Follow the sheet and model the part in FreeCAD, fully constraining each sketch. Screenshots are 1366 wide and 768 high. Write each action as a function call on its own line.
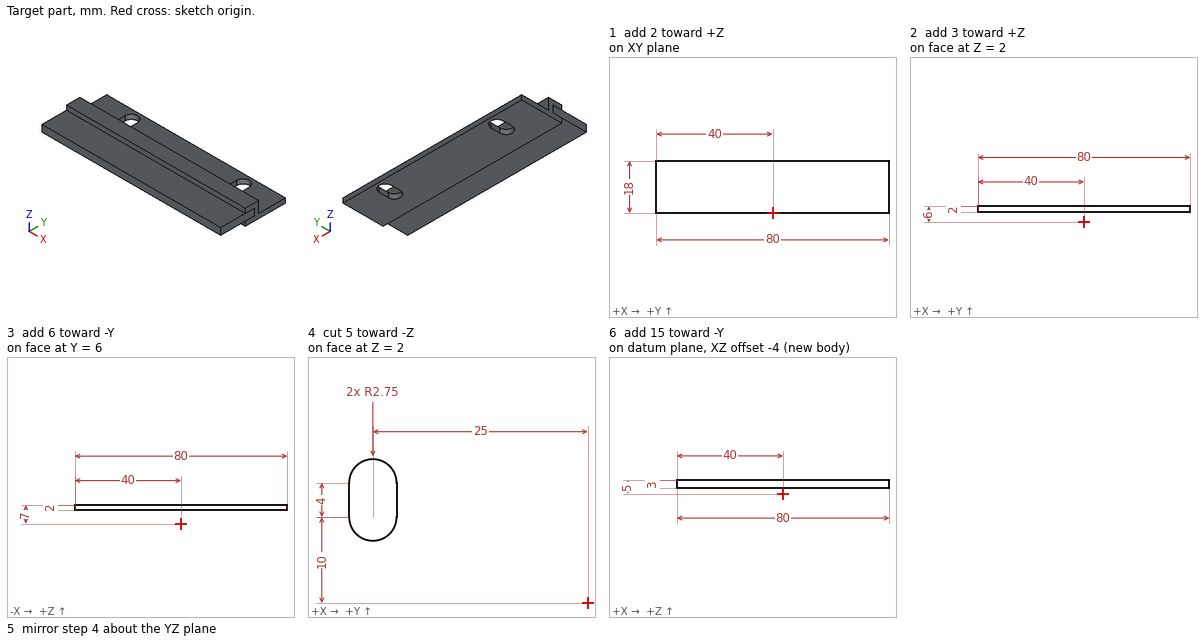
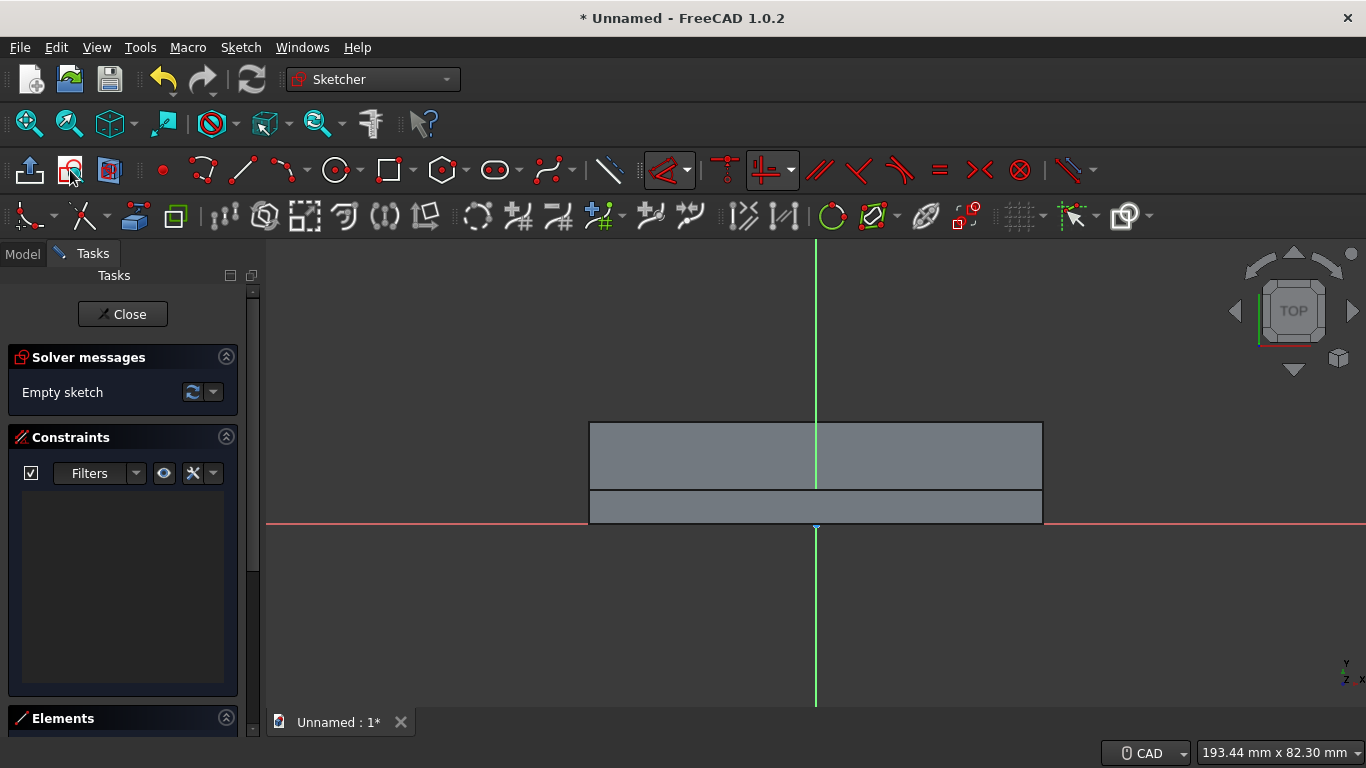
click(110, 170)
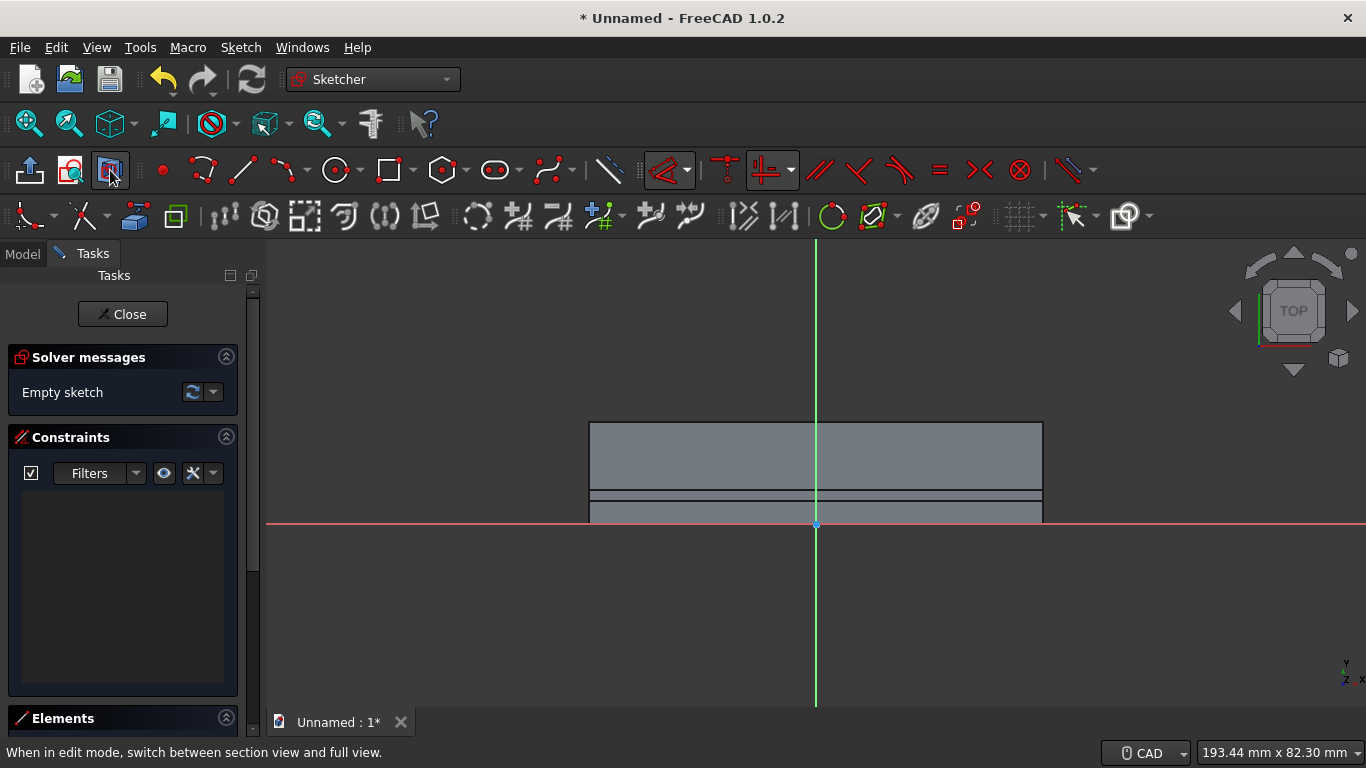
scroll(655, 452, up, 8)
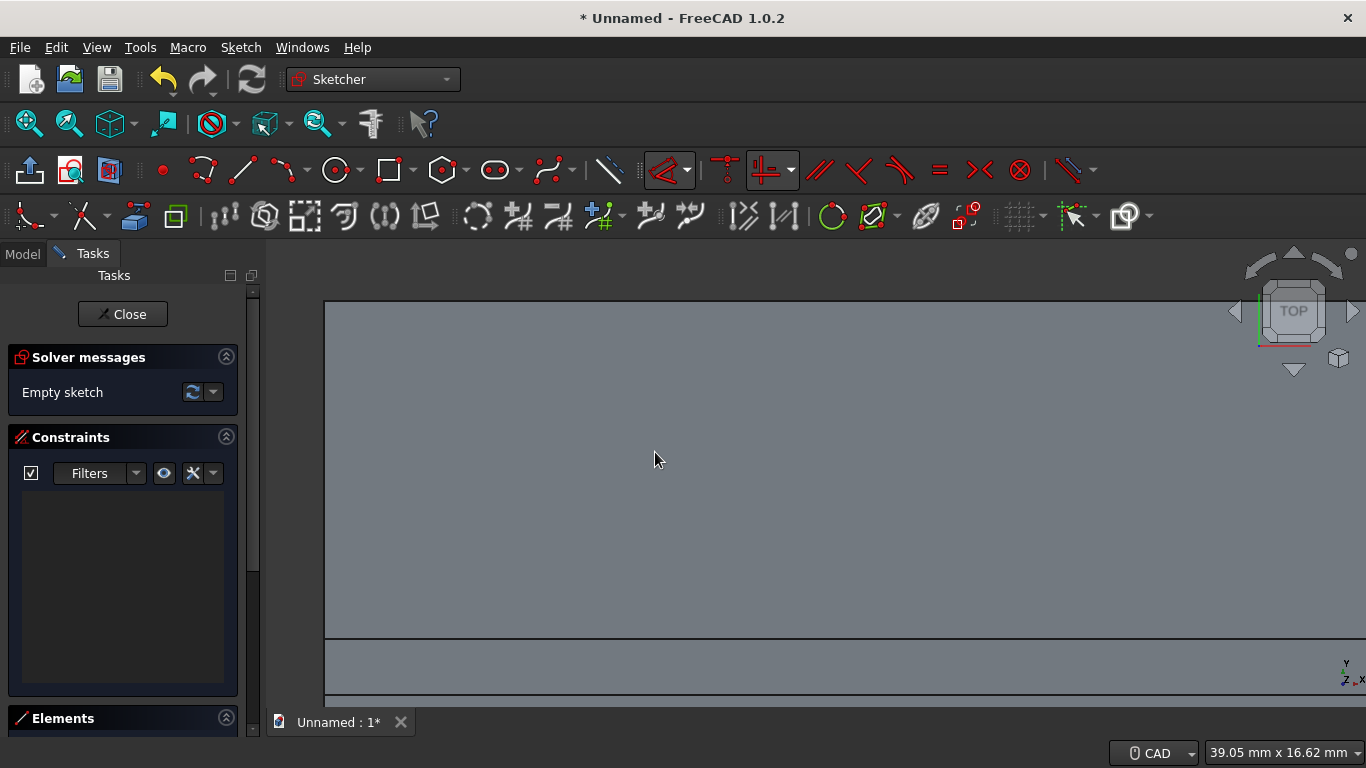
click(496, 170)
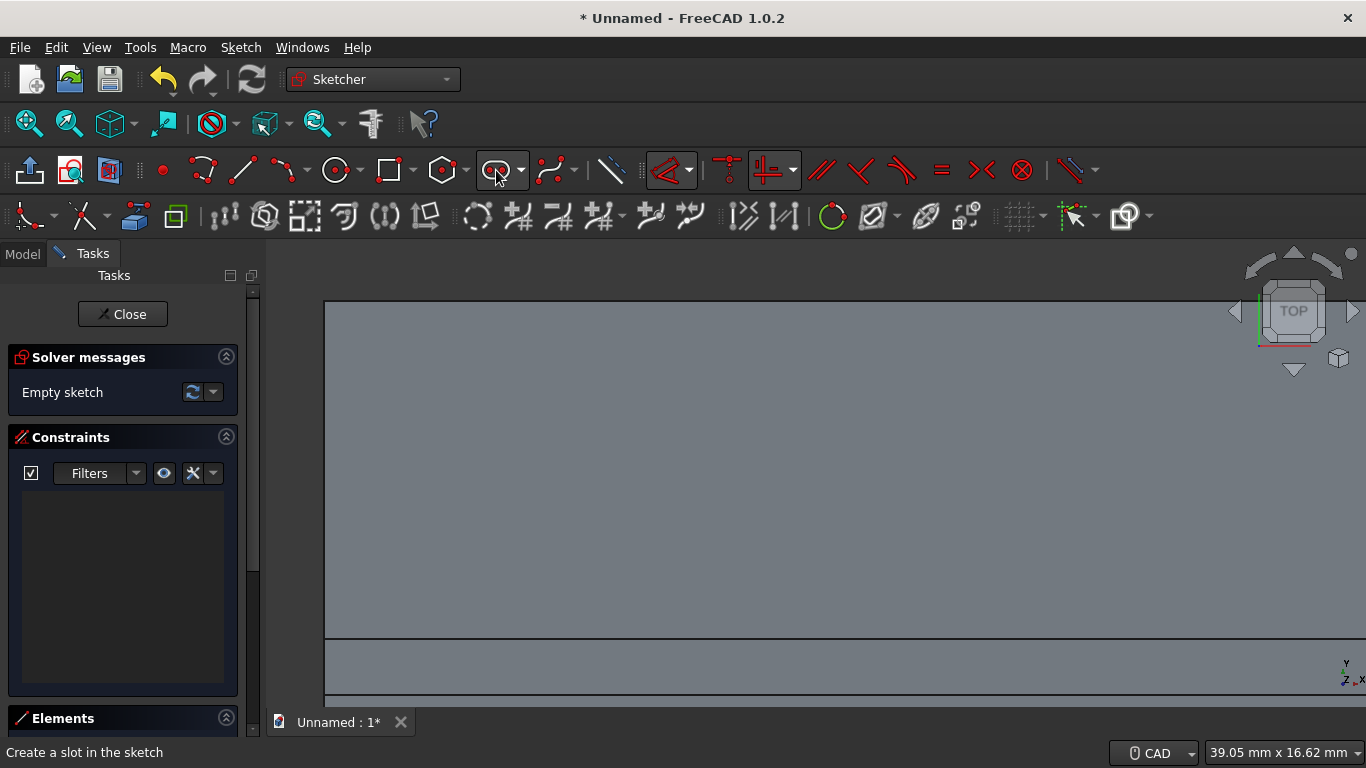
click(747, 526)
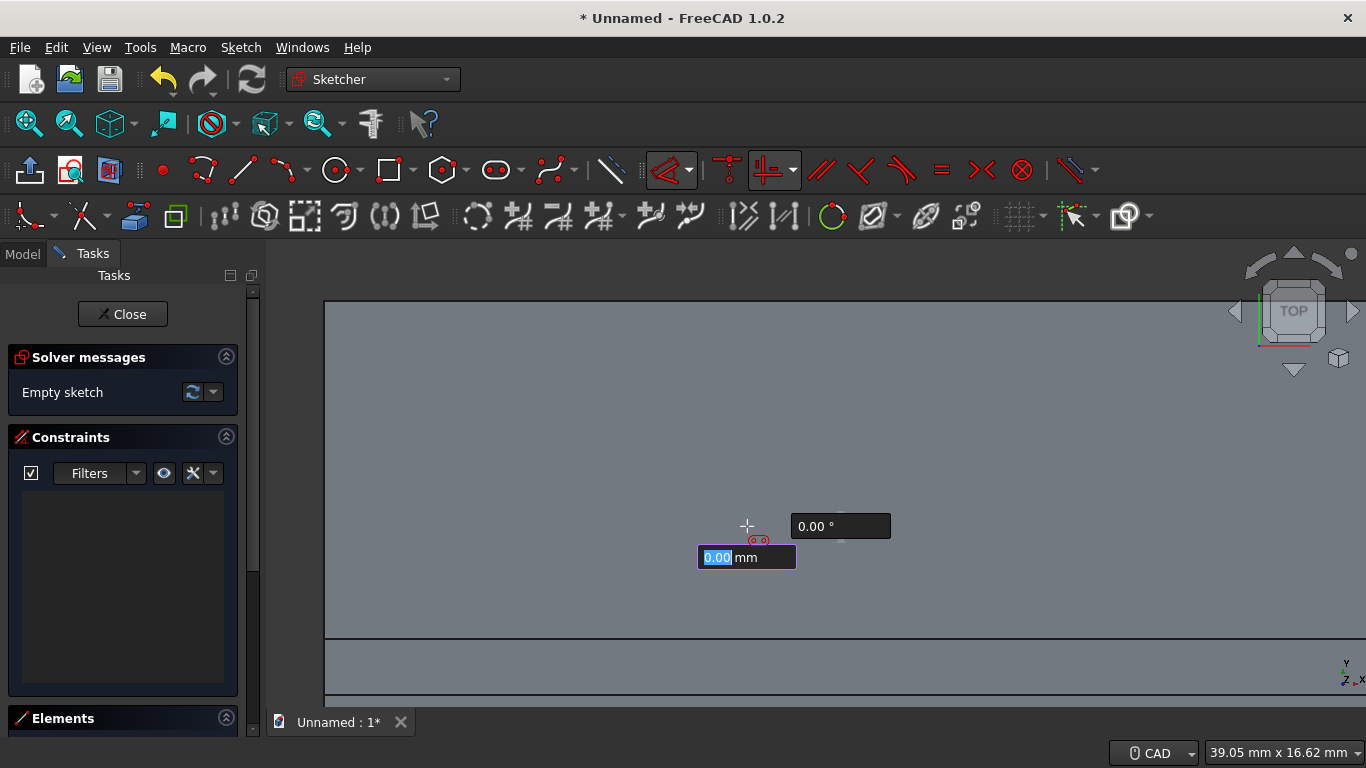
click(747, 413)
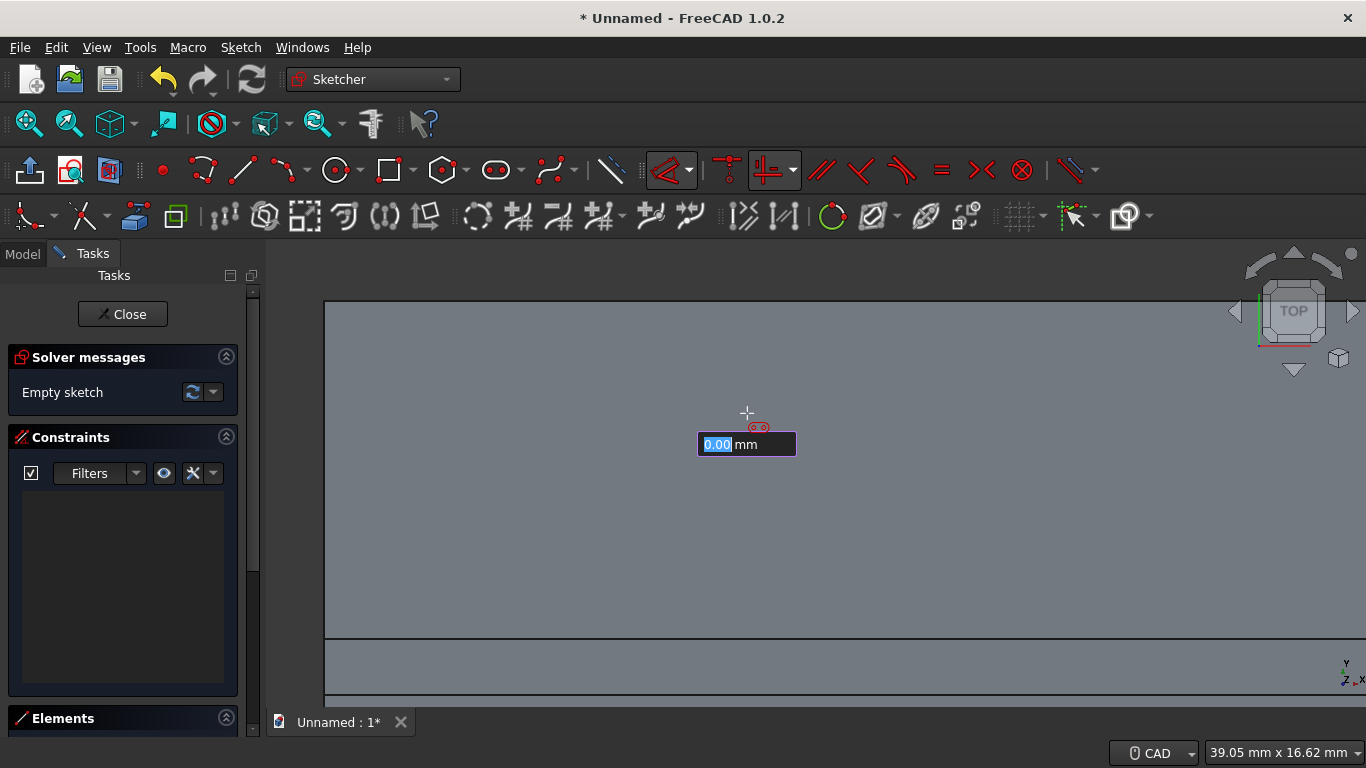
click(824, 470)
key(Escape)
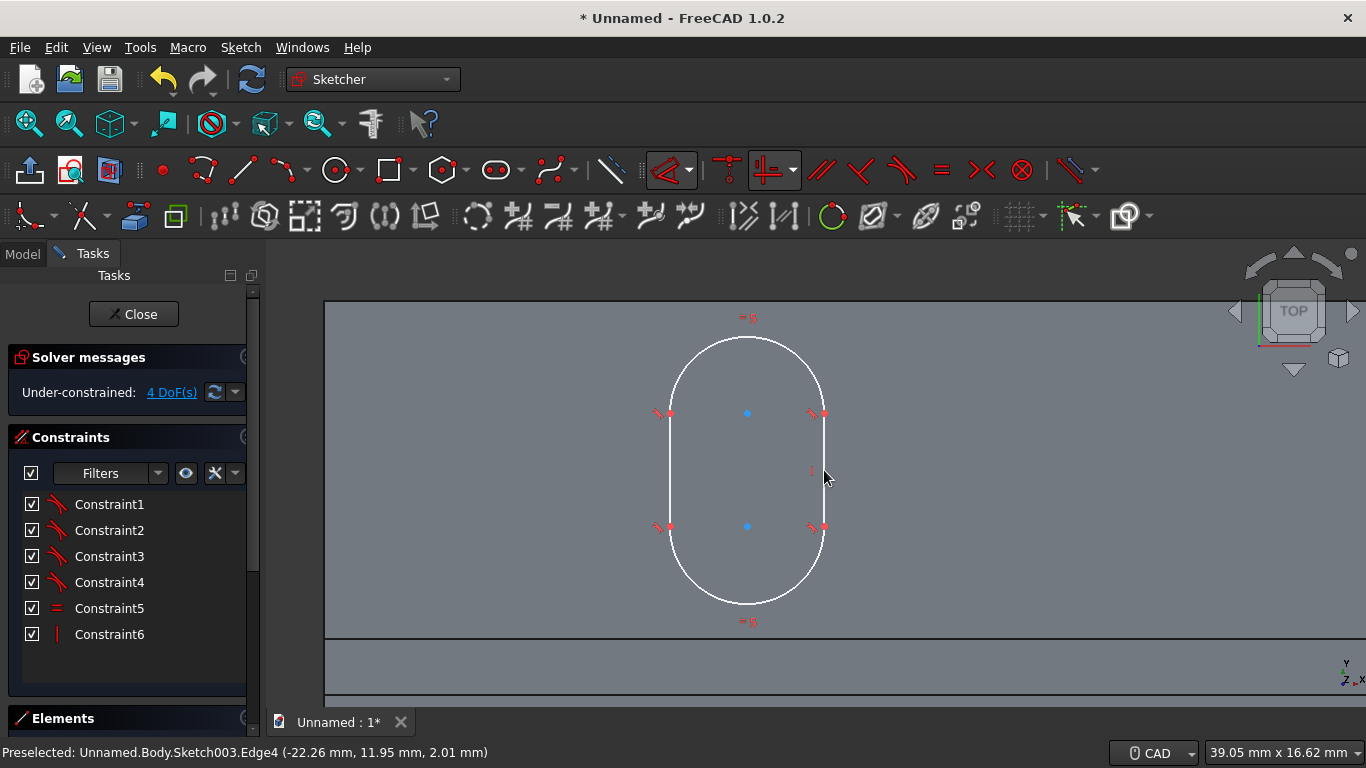
click(702, 589)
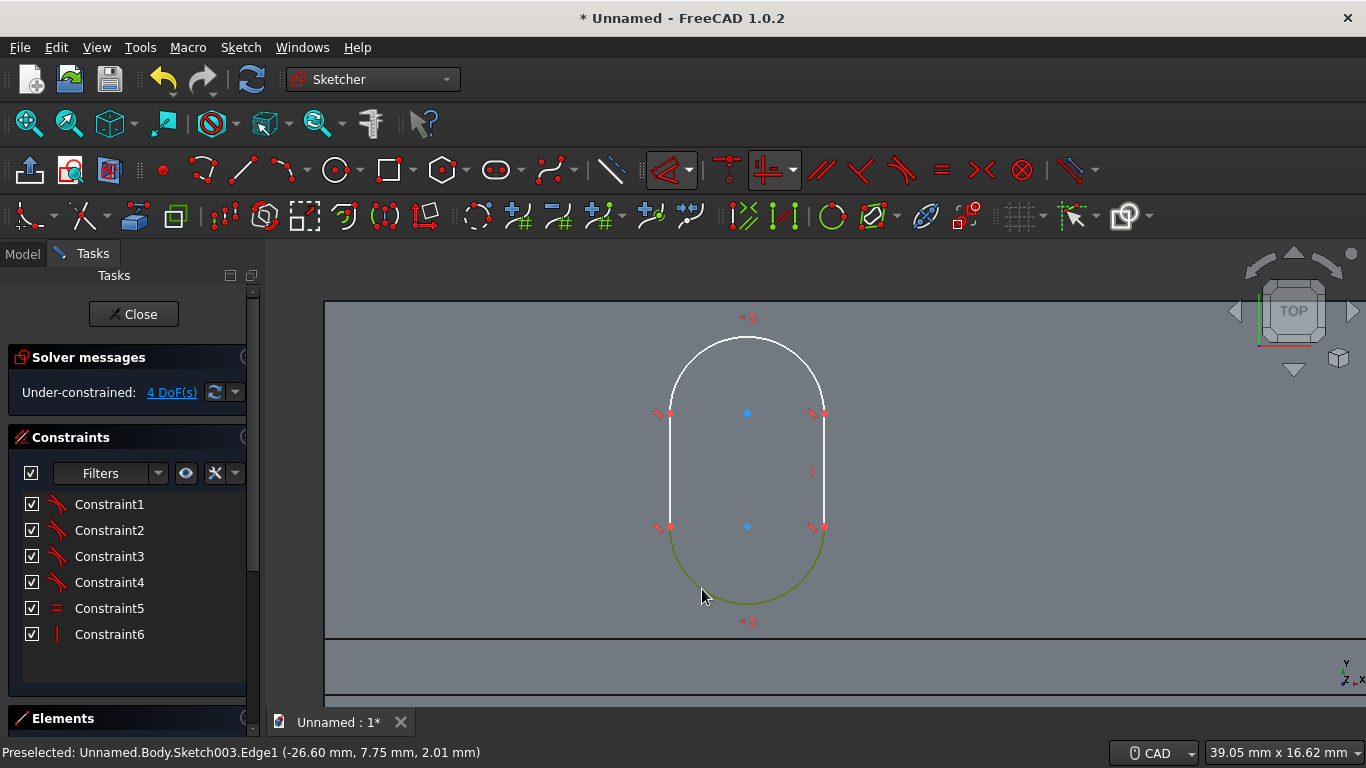
click(692, 170)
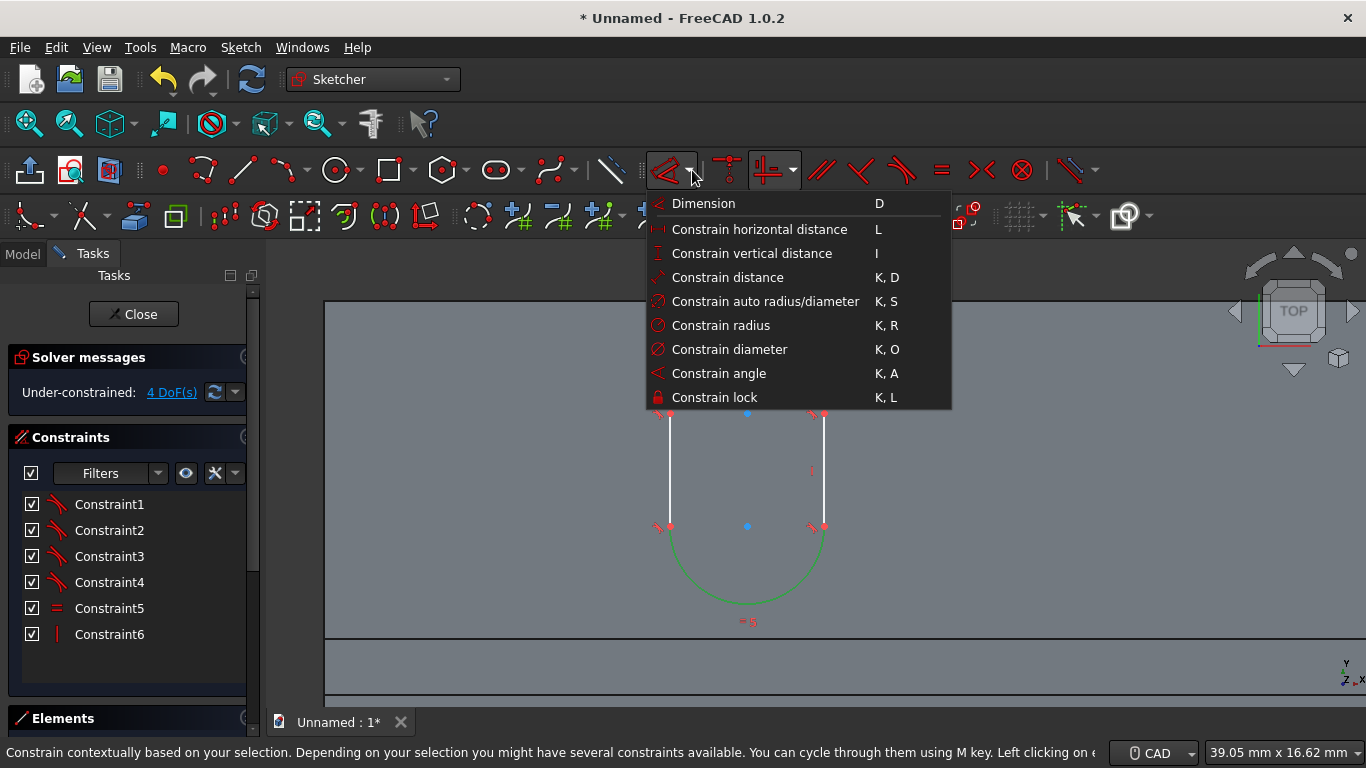
click(799, 325)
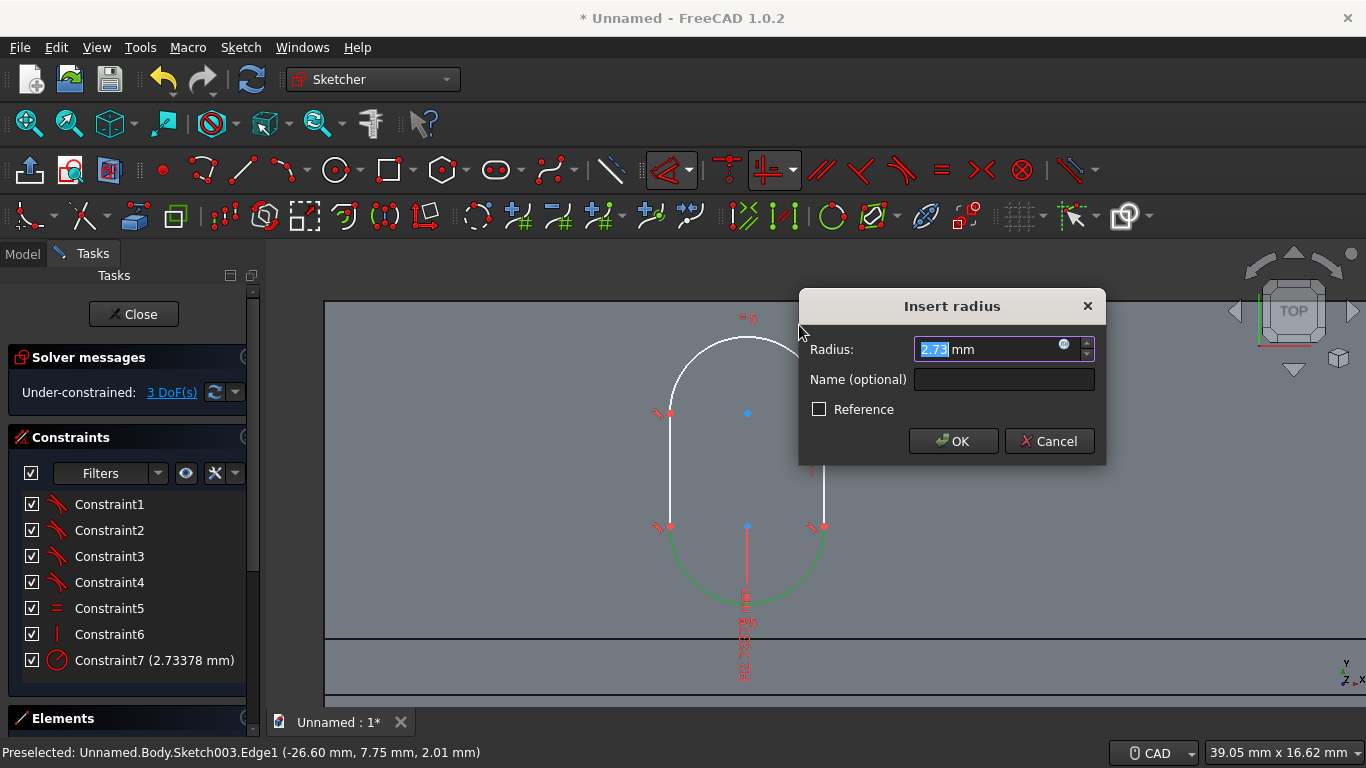
text(2.75)
key(Return)